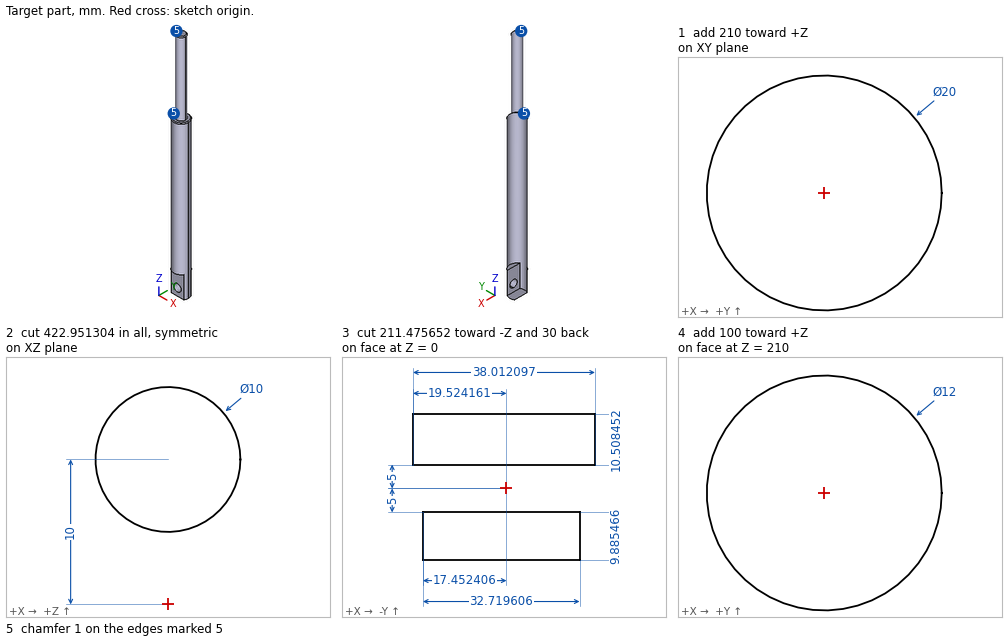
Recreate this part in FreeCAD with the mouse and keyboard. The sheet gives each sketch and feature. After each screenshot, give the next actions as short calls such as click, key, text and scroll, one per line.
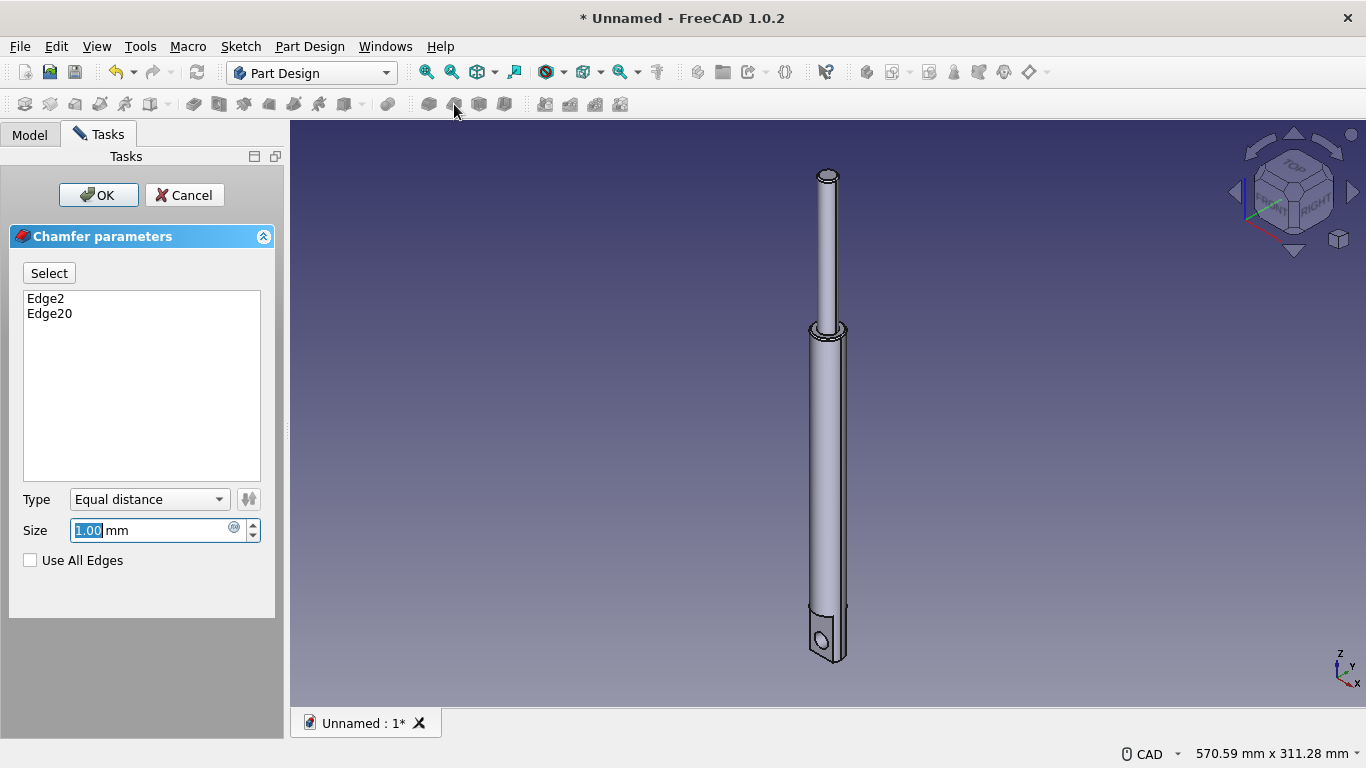
text(1)
key(Tab)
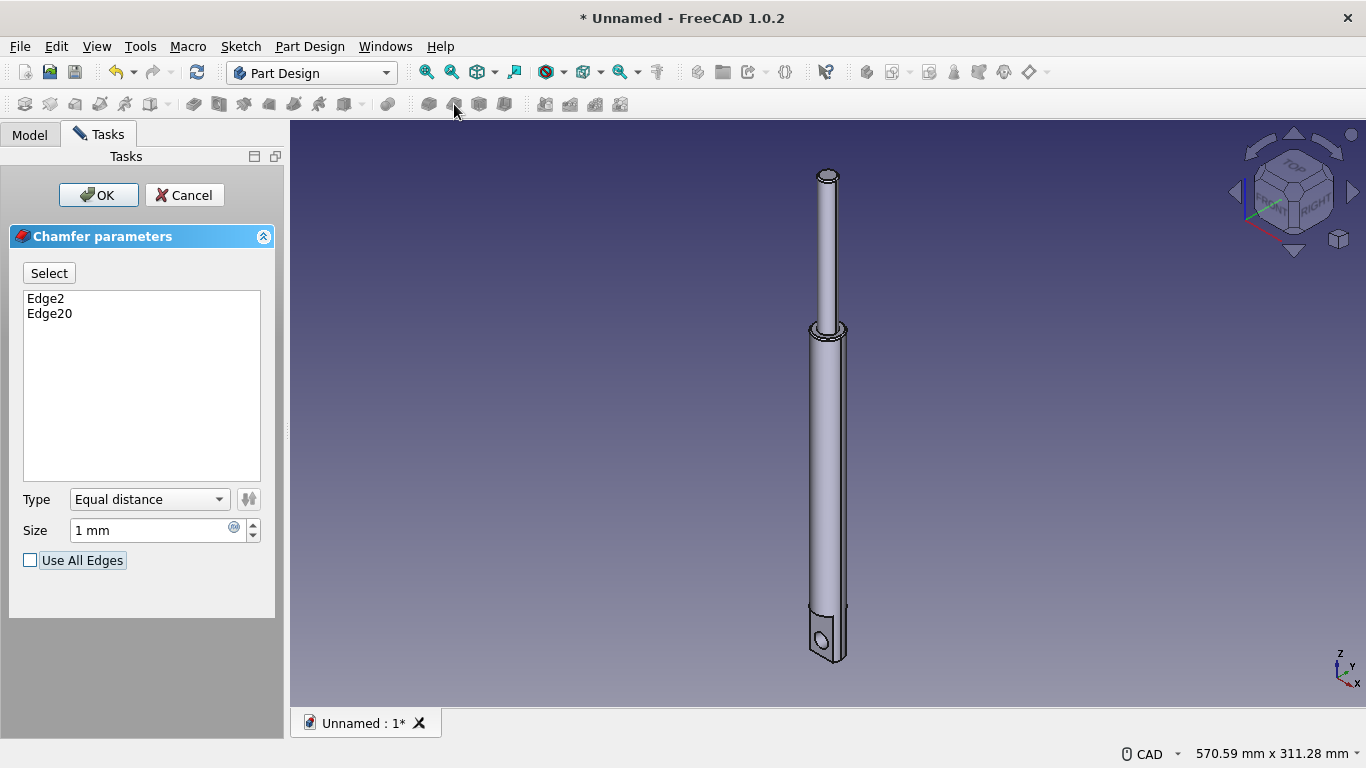
click(99, 195)